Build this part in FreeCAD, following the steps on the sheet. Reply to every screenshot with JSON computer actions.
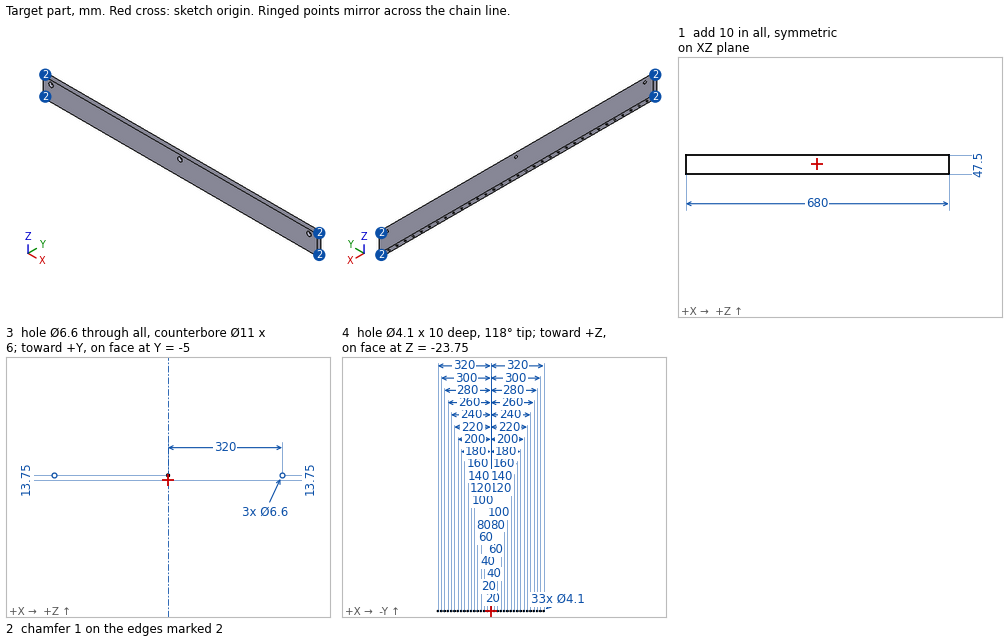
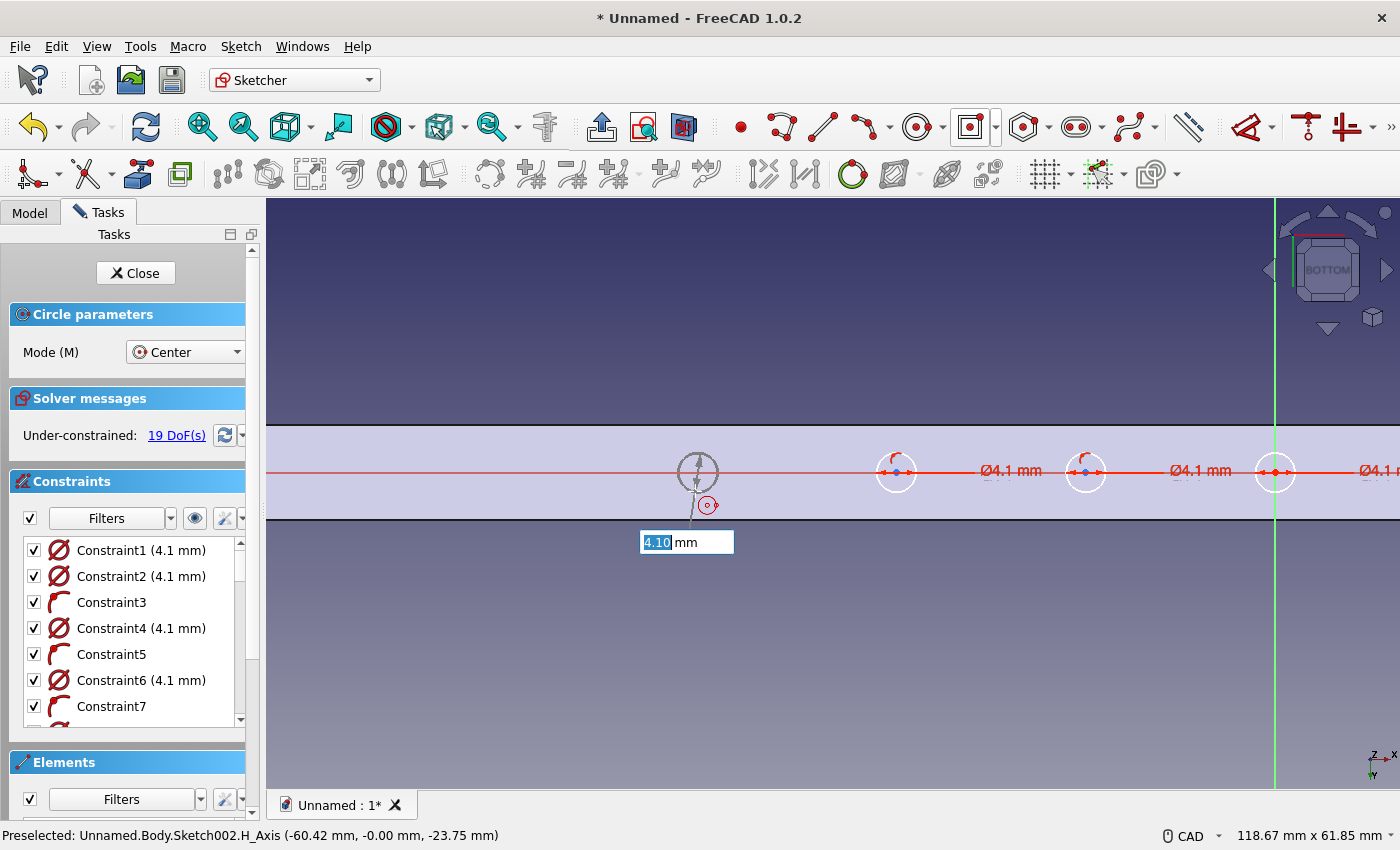
{"action": "type", "text": "4.1"}
{"action": "key", "text": "Return"}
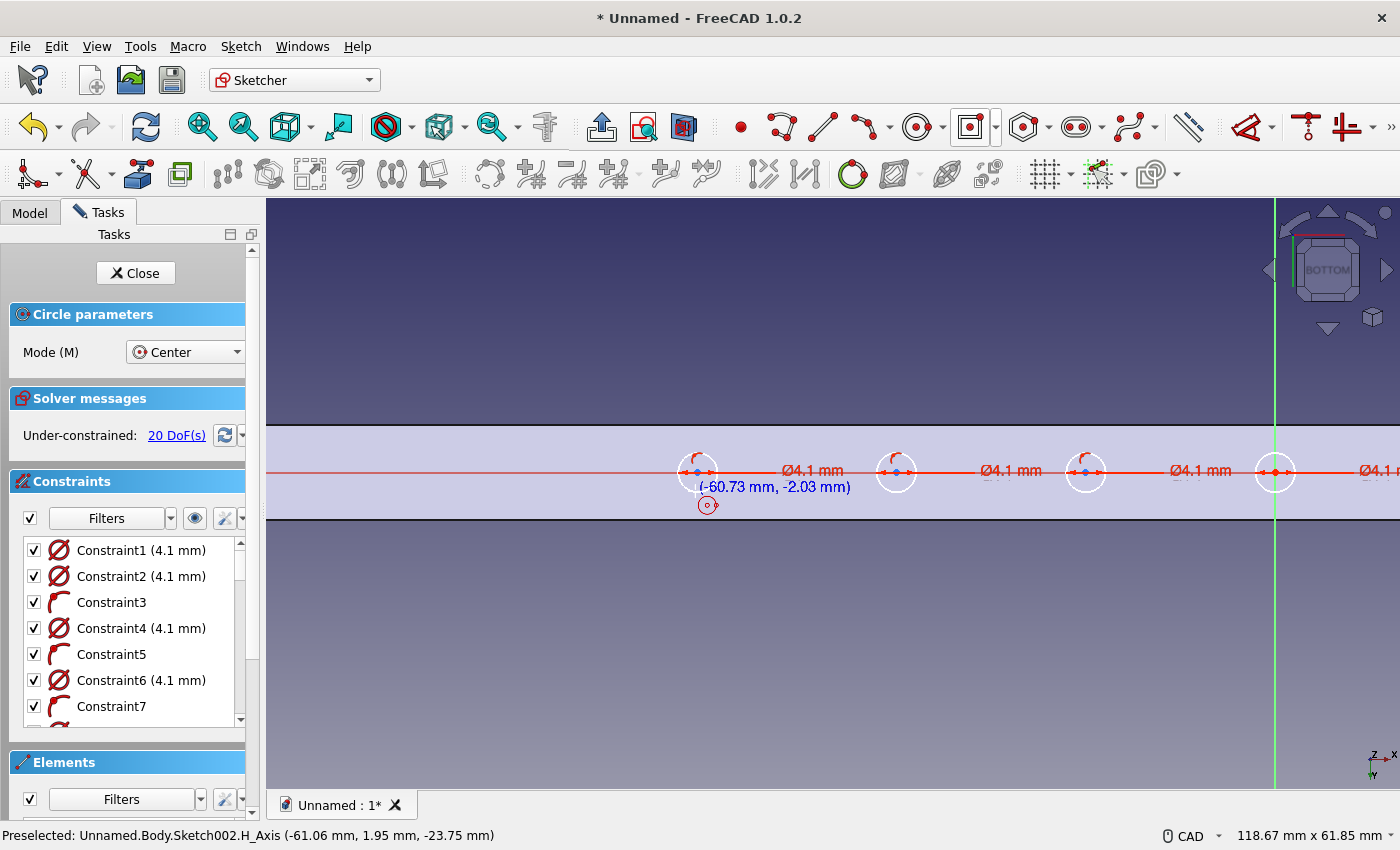
{"action": "scroll", "coordinate": [701, 496], "scroll_direction": "down", "scroll_amount": 11}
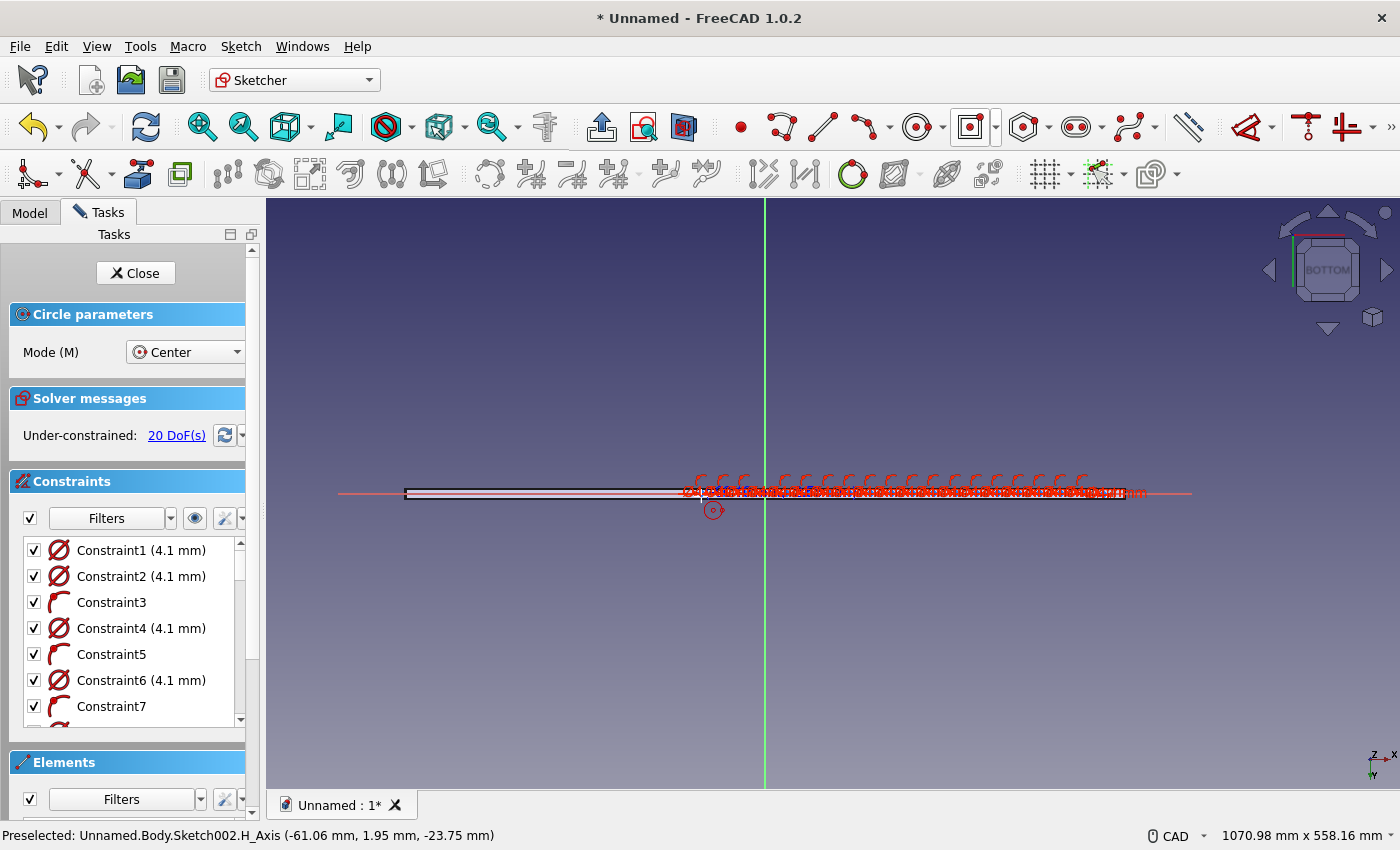
{"action": "left_click", "coordinate": [680, 494]}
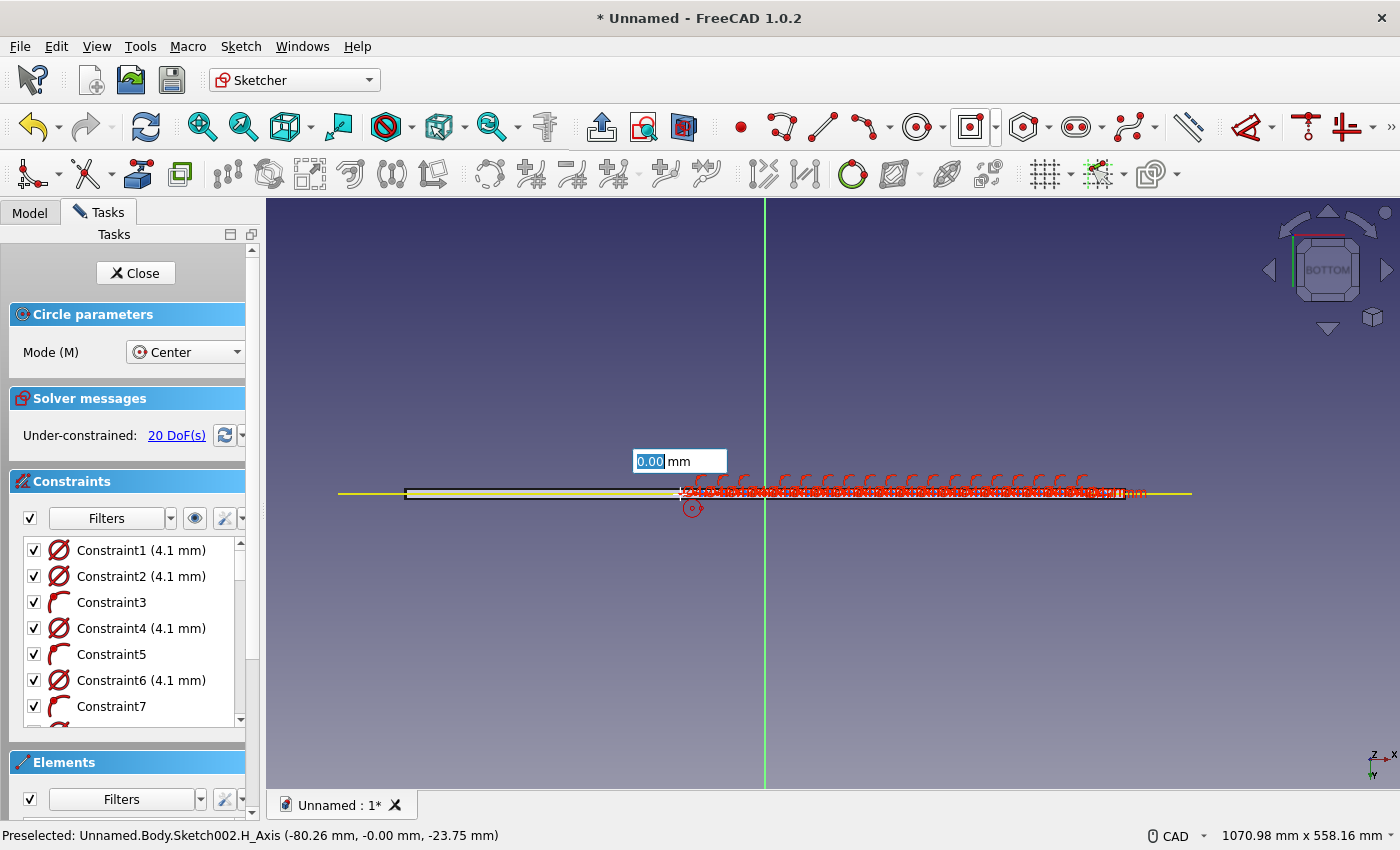
{"action": "scroll", "coordinate": [681, 492], "scroll_direction": "up", "scroll_amount": 11}
{"action": "mouse_move", "coordinate": [678, 486]}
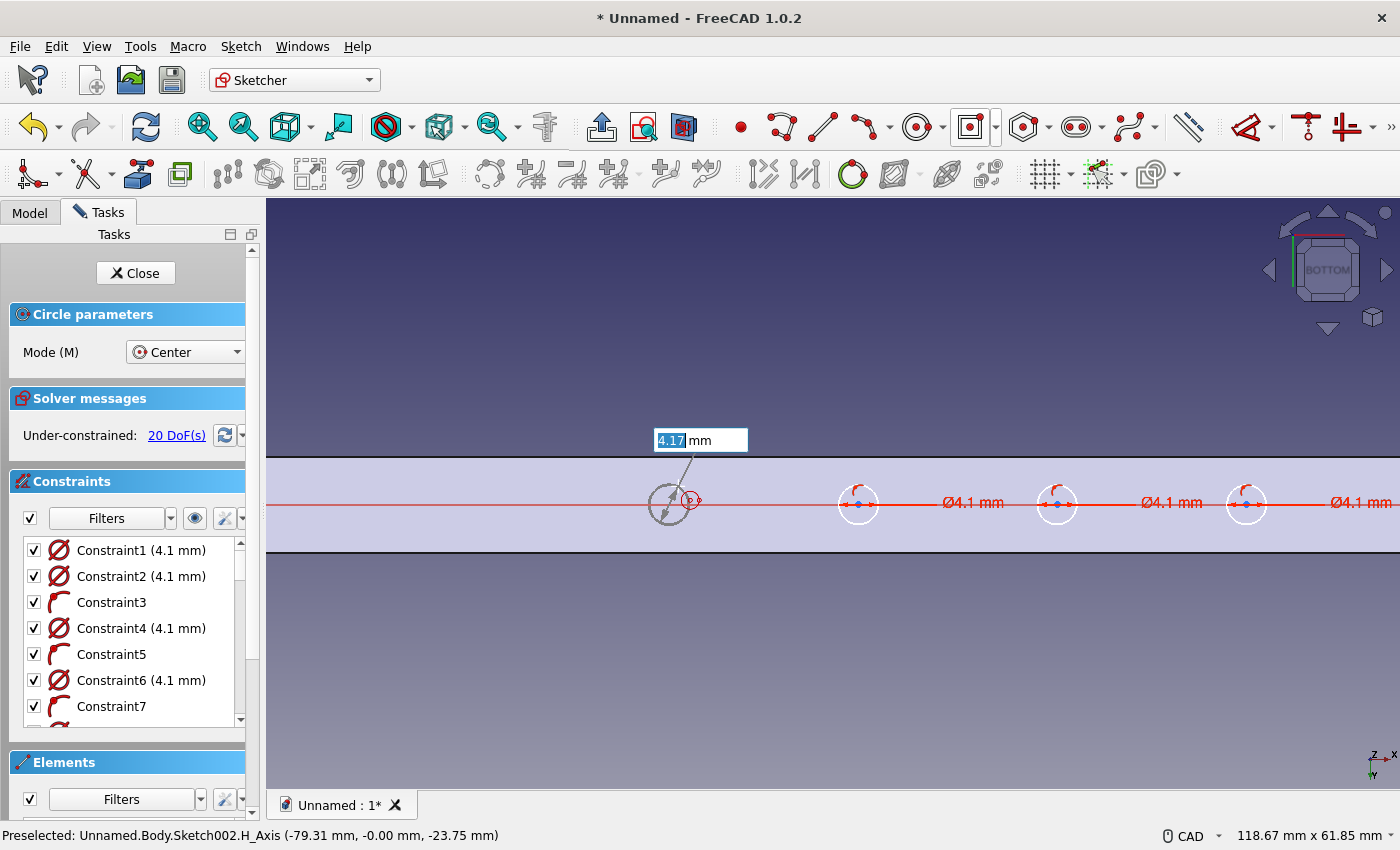
{"action": "type", "text": "4.1"}
{"action": "key", "text": "Return"}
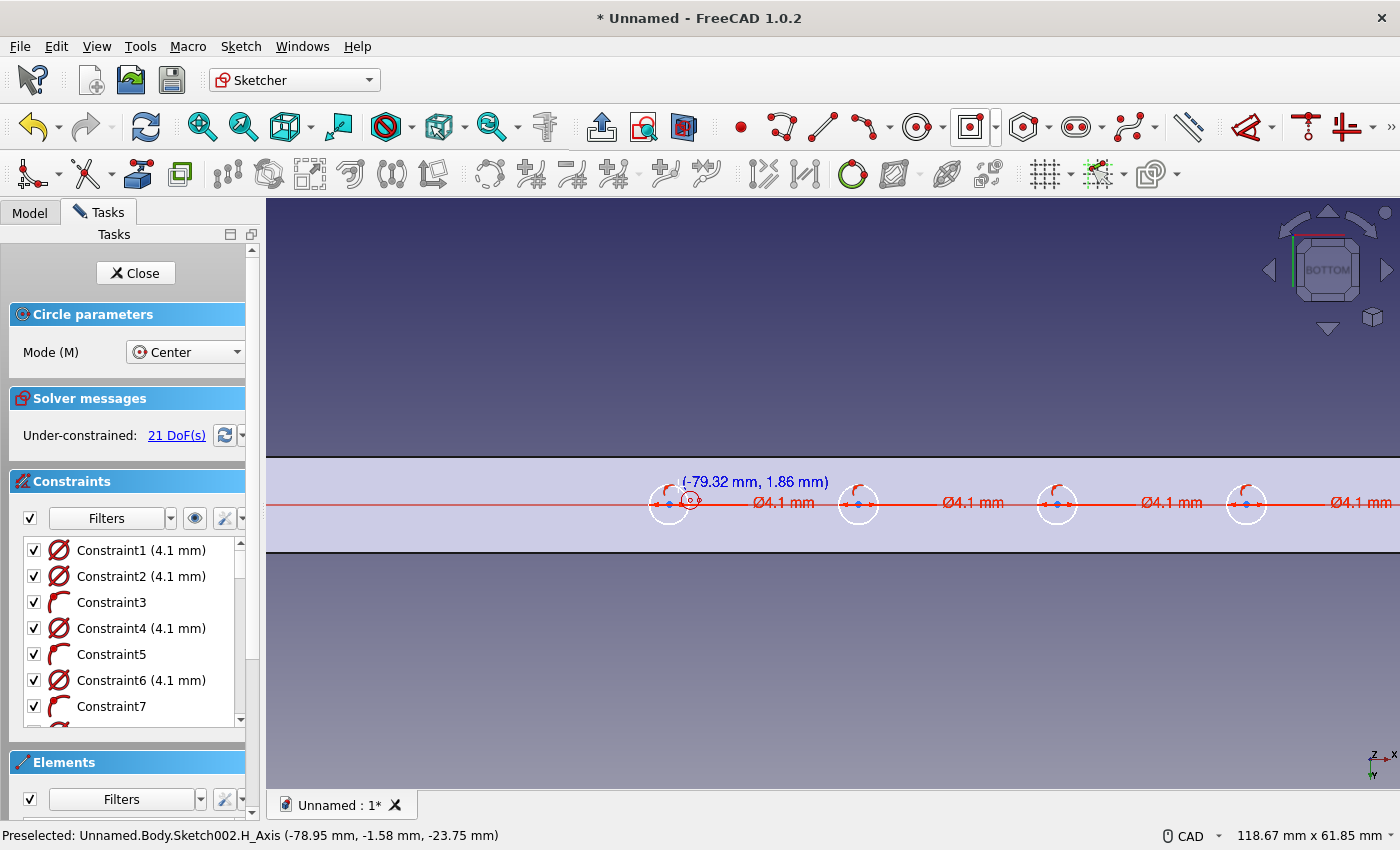
{"action": "scroll", "coordinate": [681, 492], "scroll_direction": "down", "scroll_amount": 11}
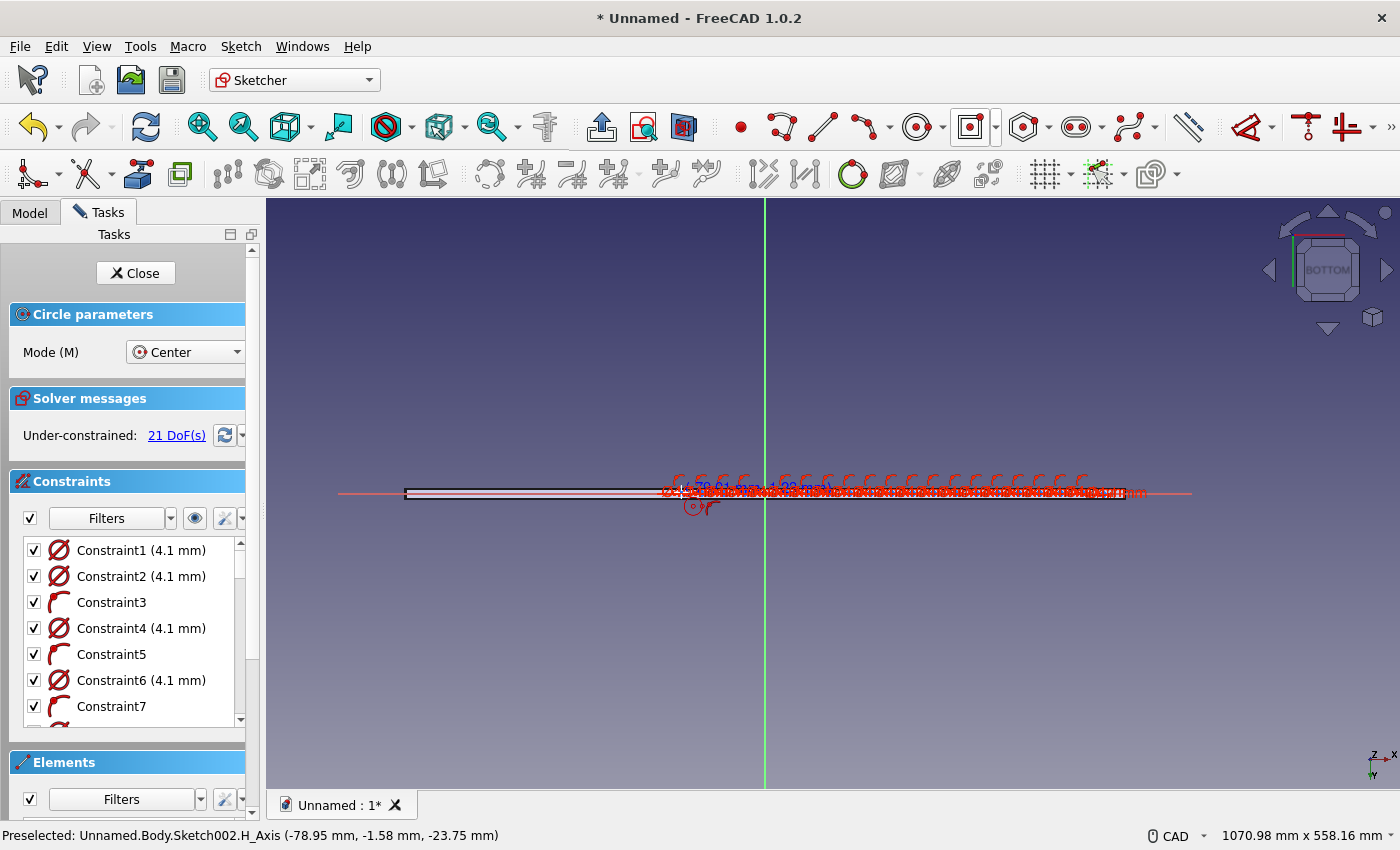
{"action": "left_click", "coordinate": [659, 494]}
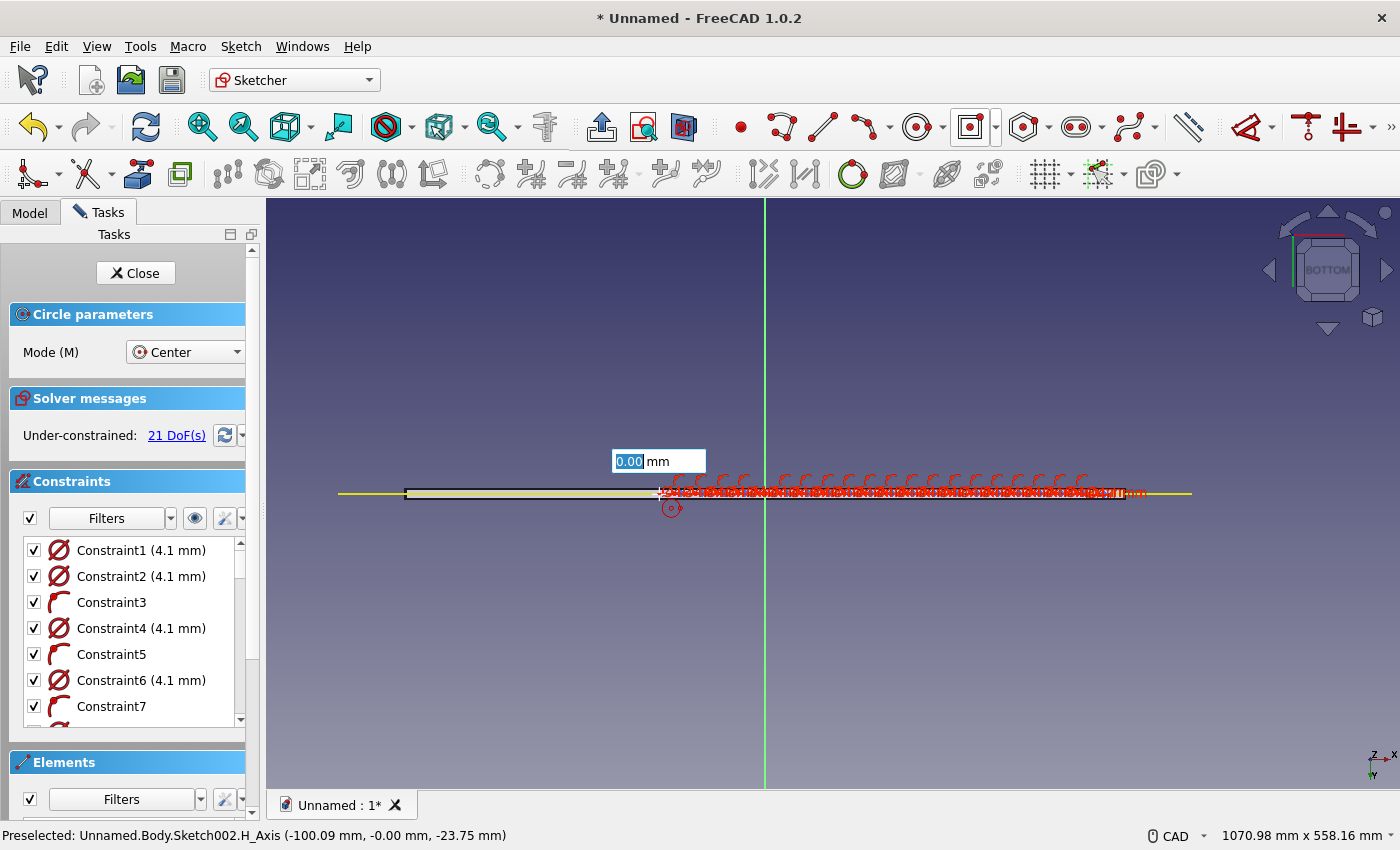
{"action": "scroll", "coordinate": [660, 492], "scroll_direction": "up", "scroll_amount": 11}
{"action": "mouse_move", "coordinate": [656, 486]}